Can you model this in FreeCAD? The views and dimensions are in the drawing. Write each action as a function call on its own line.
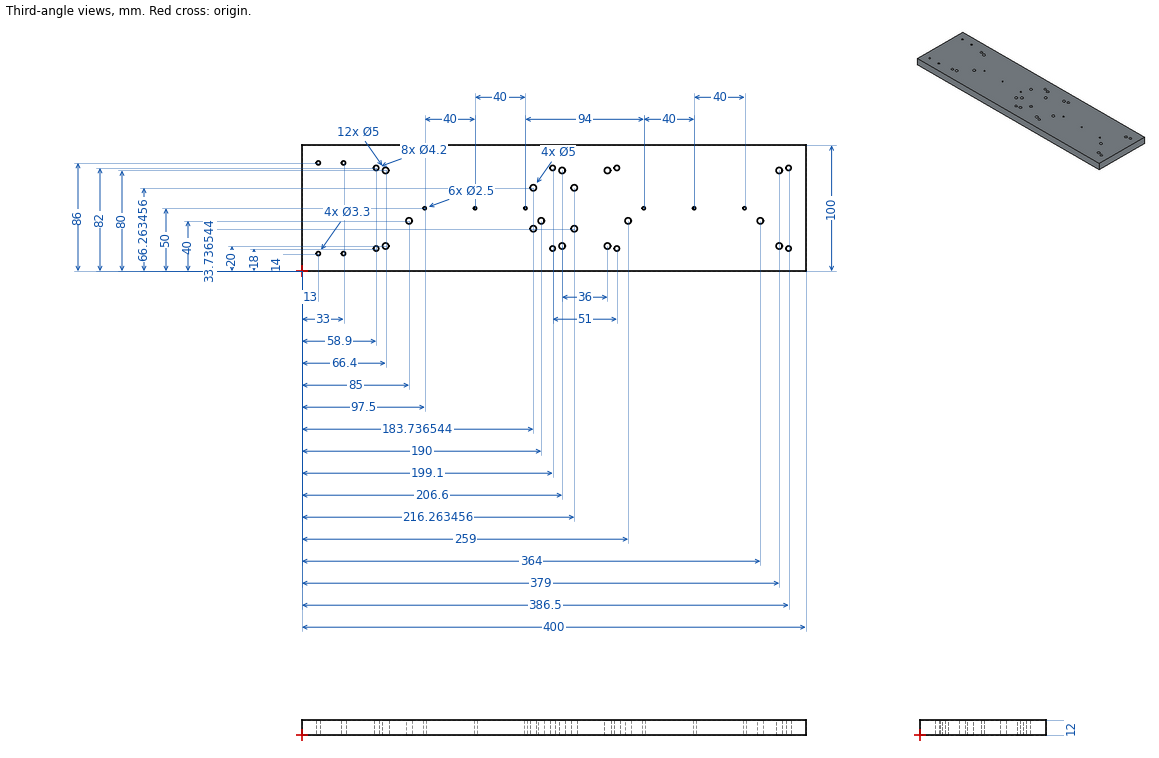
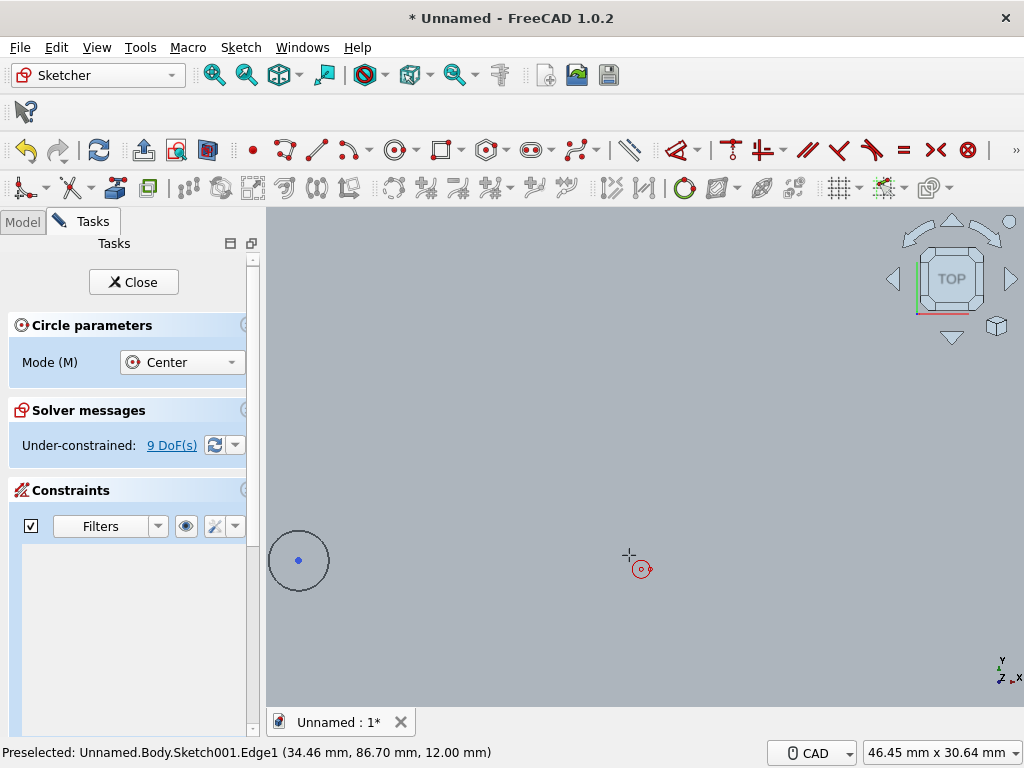
scroll(629, 556, down, 8)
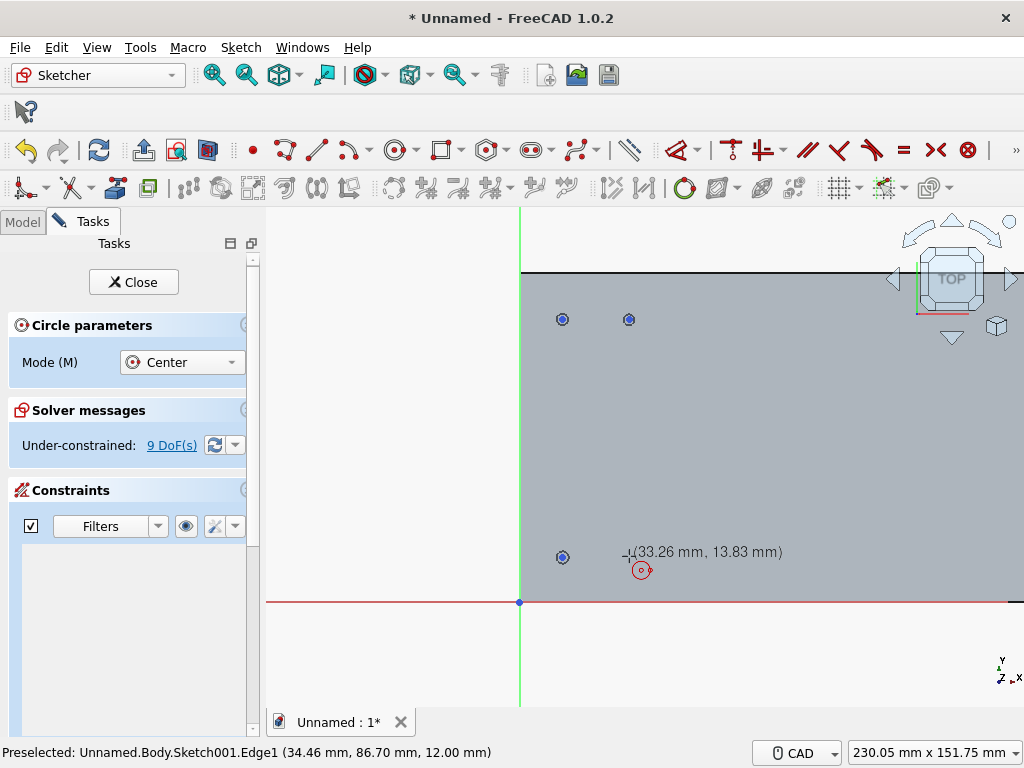
click(629, 556)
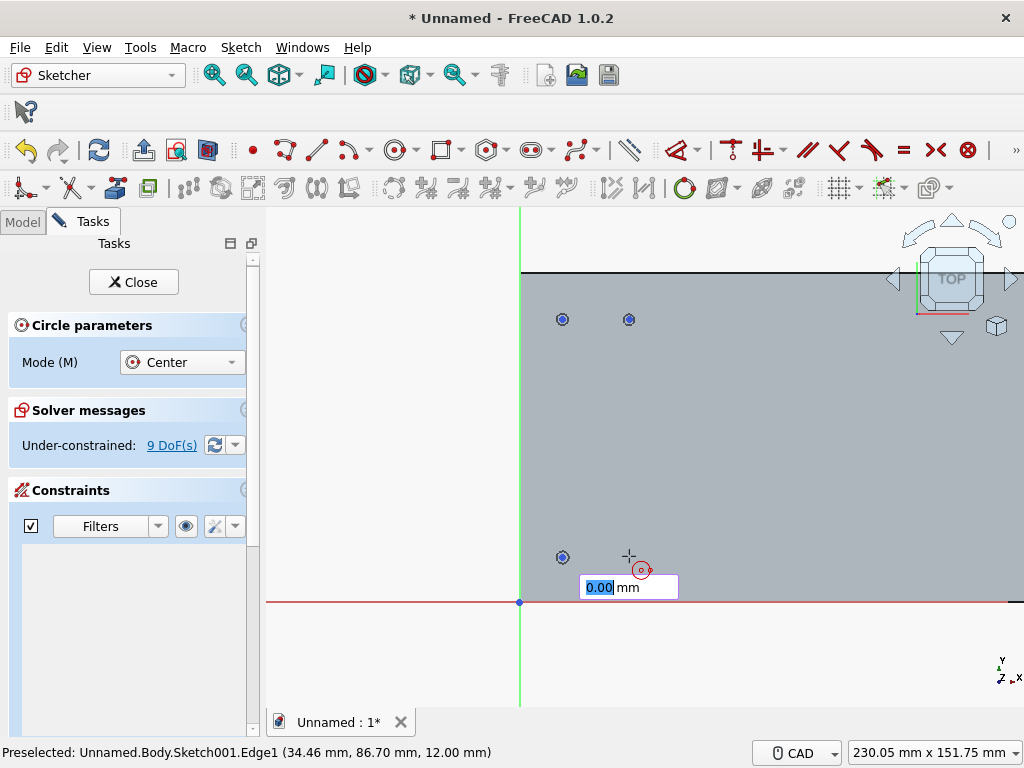
scroll(632, 552, up, 6)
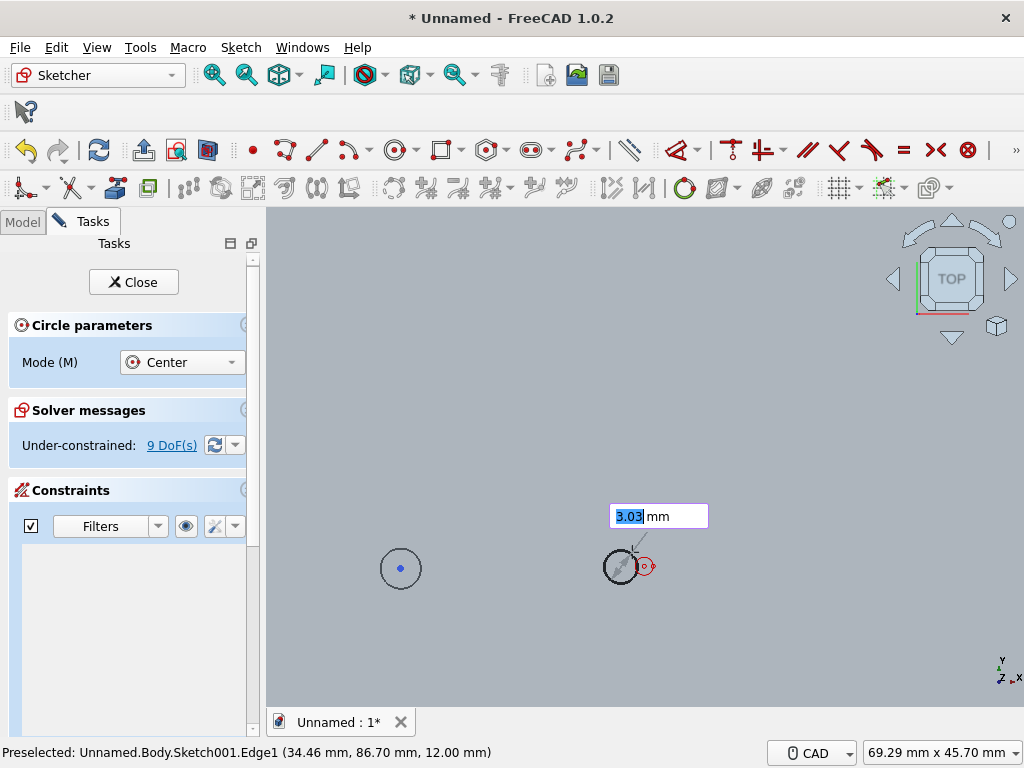
click(632, 552)
key(Escape)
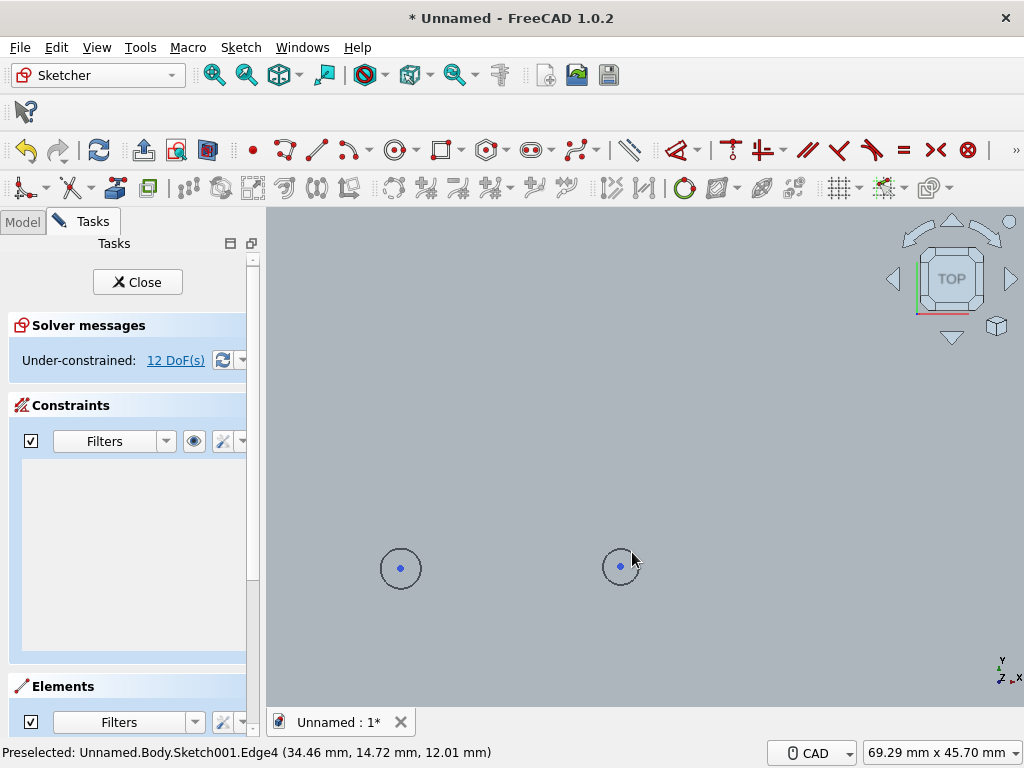
click(415, 554)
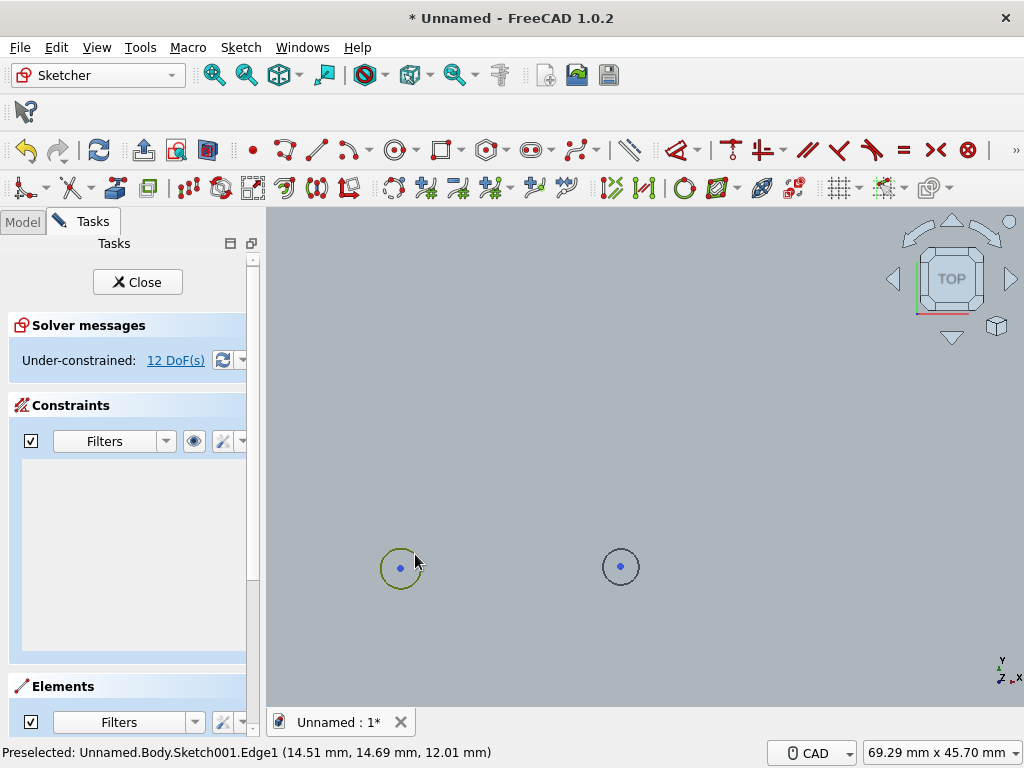
scroll(632, 551, down, 6)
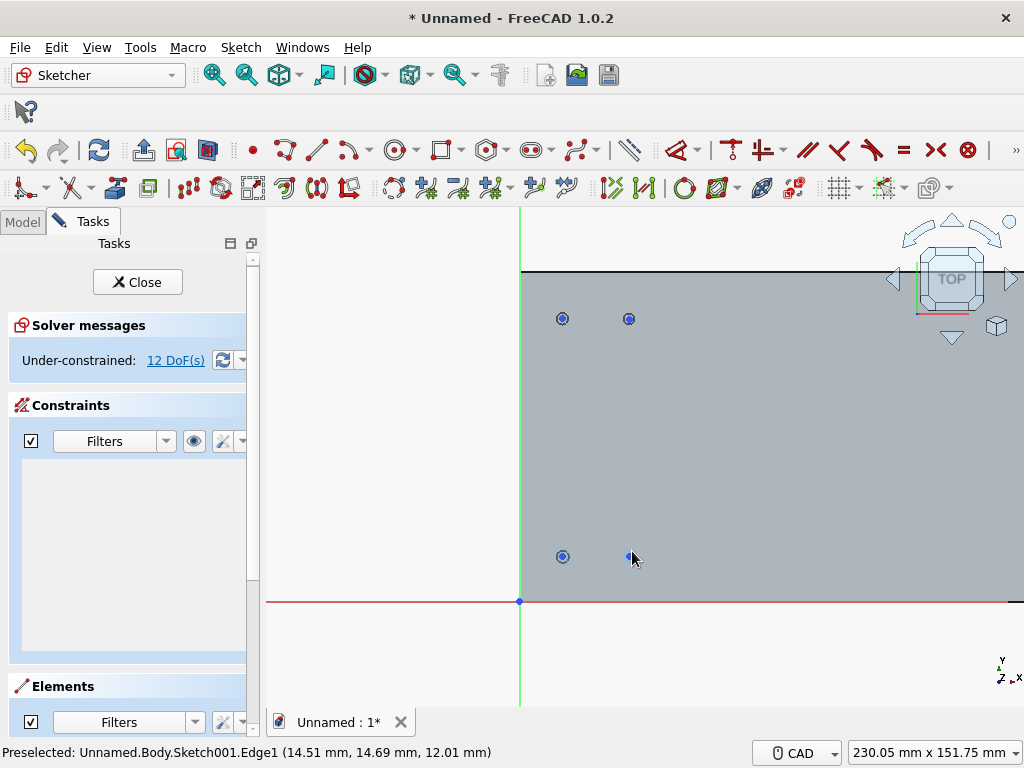
scroll(566, 315, up, 5)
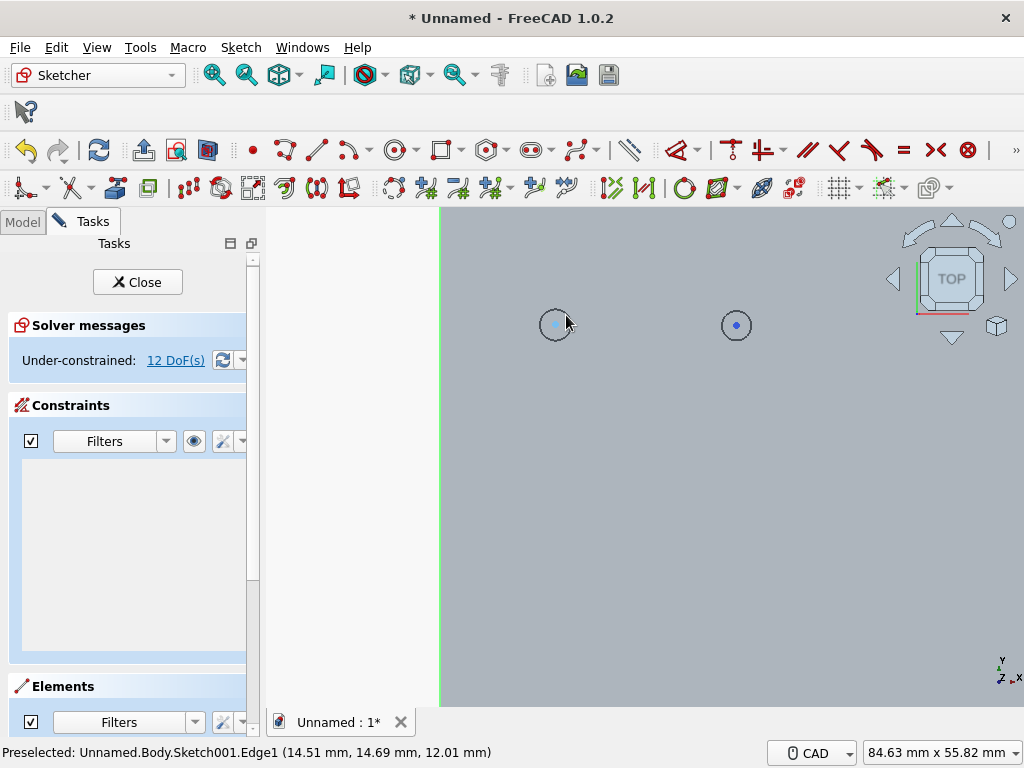
click(567, 314)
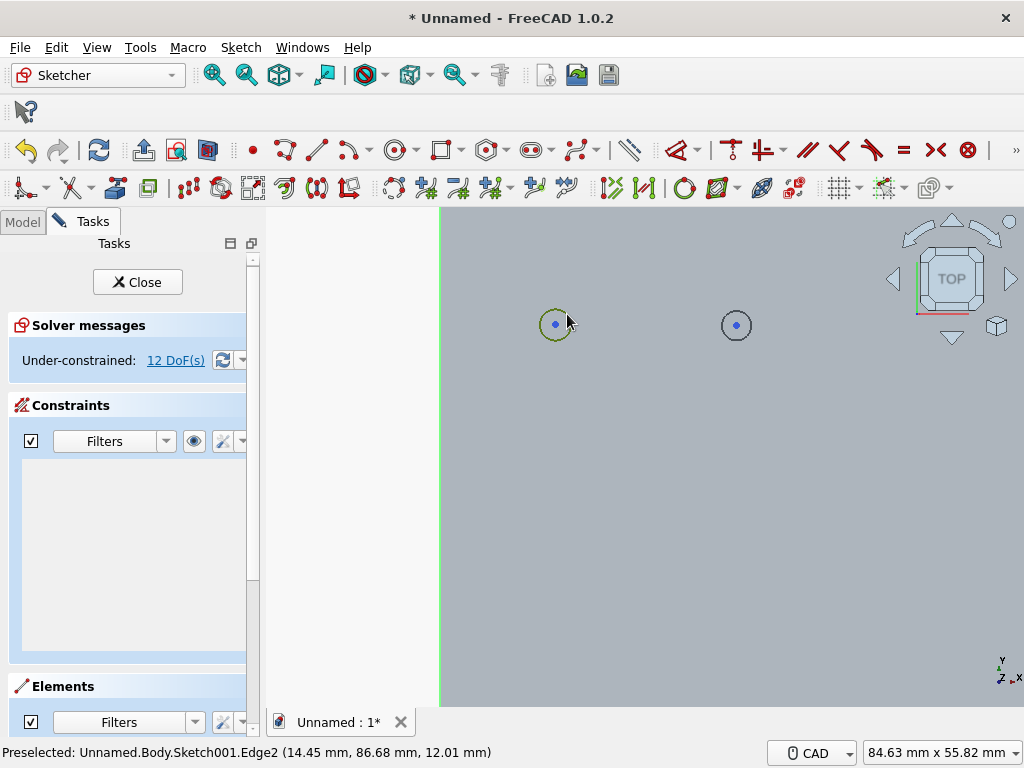
click(747, 315)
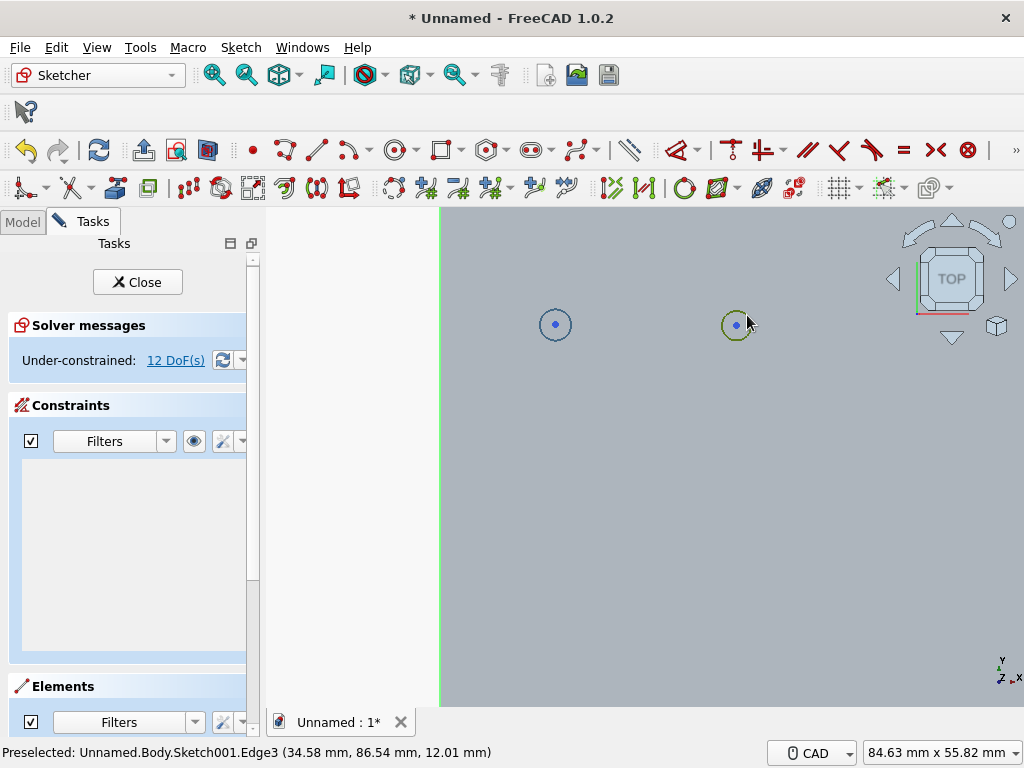
scroll(566, 315, down, 5)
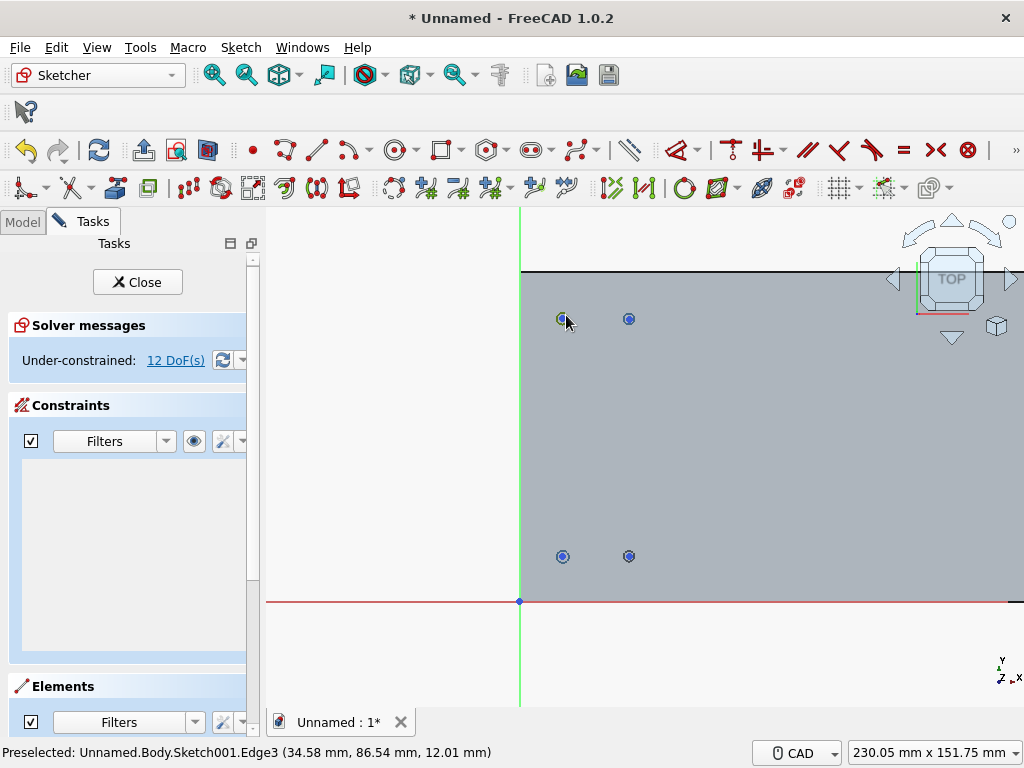
scroll(633, 552, up, 5)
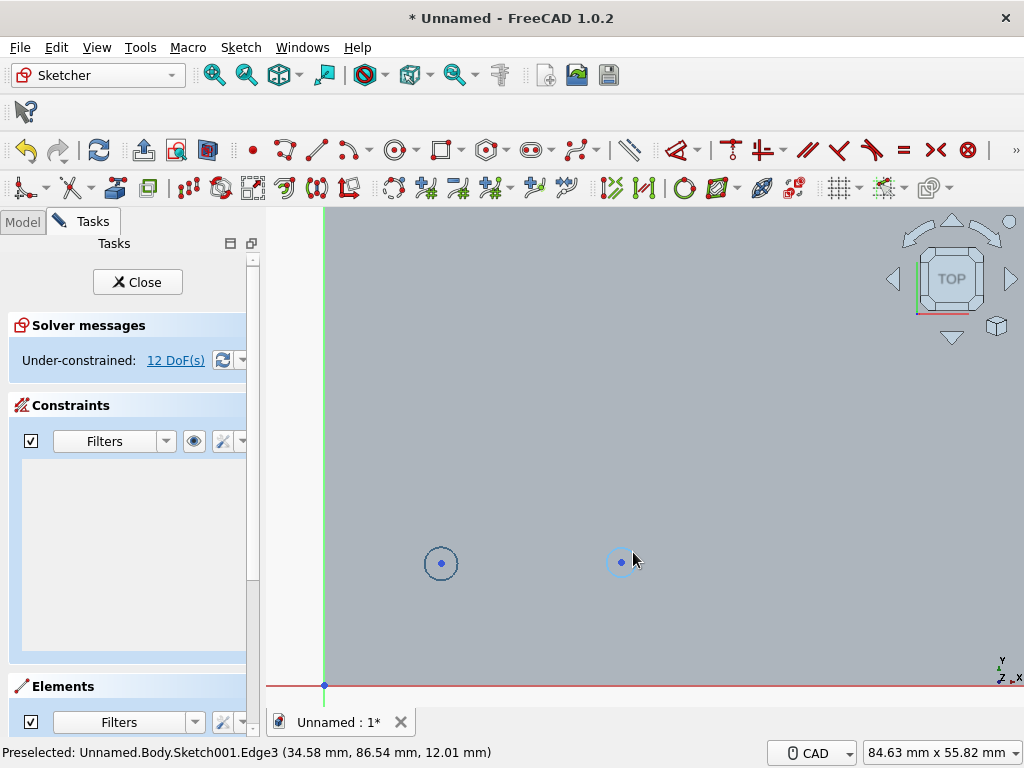
click(632, 552)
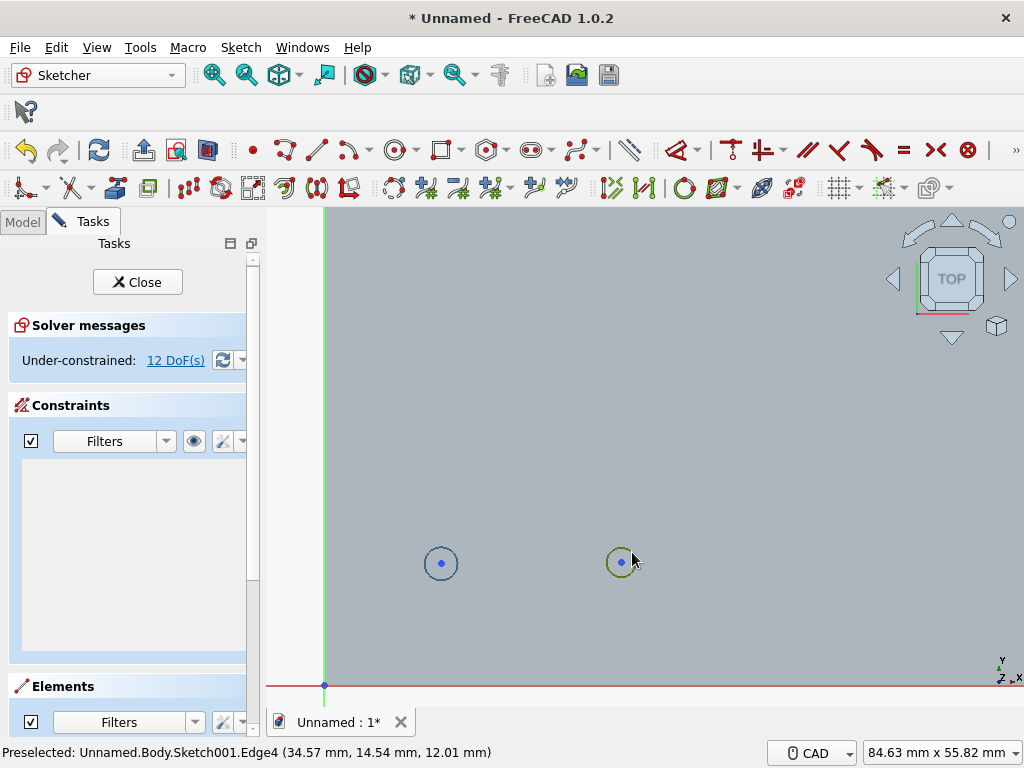
click(904, 150)